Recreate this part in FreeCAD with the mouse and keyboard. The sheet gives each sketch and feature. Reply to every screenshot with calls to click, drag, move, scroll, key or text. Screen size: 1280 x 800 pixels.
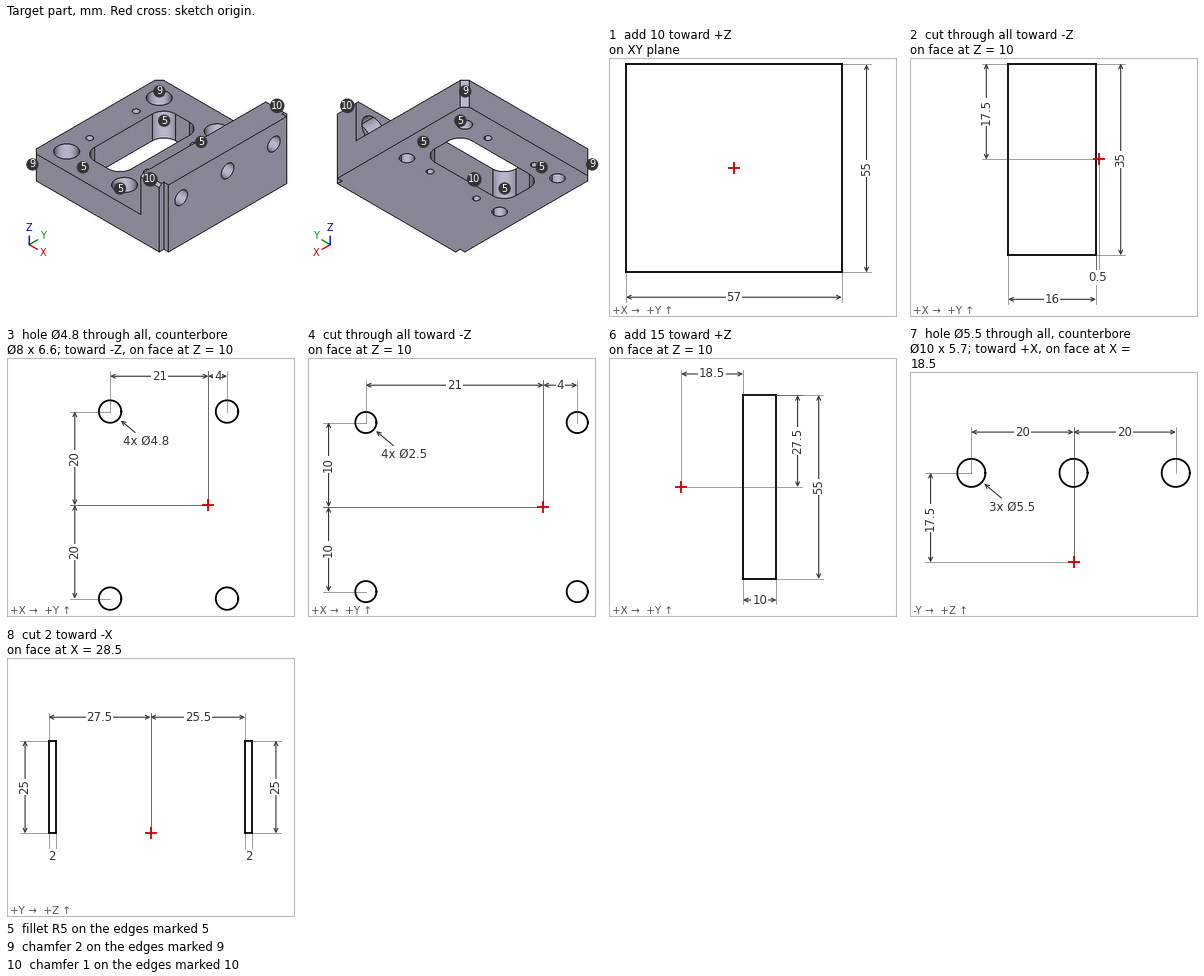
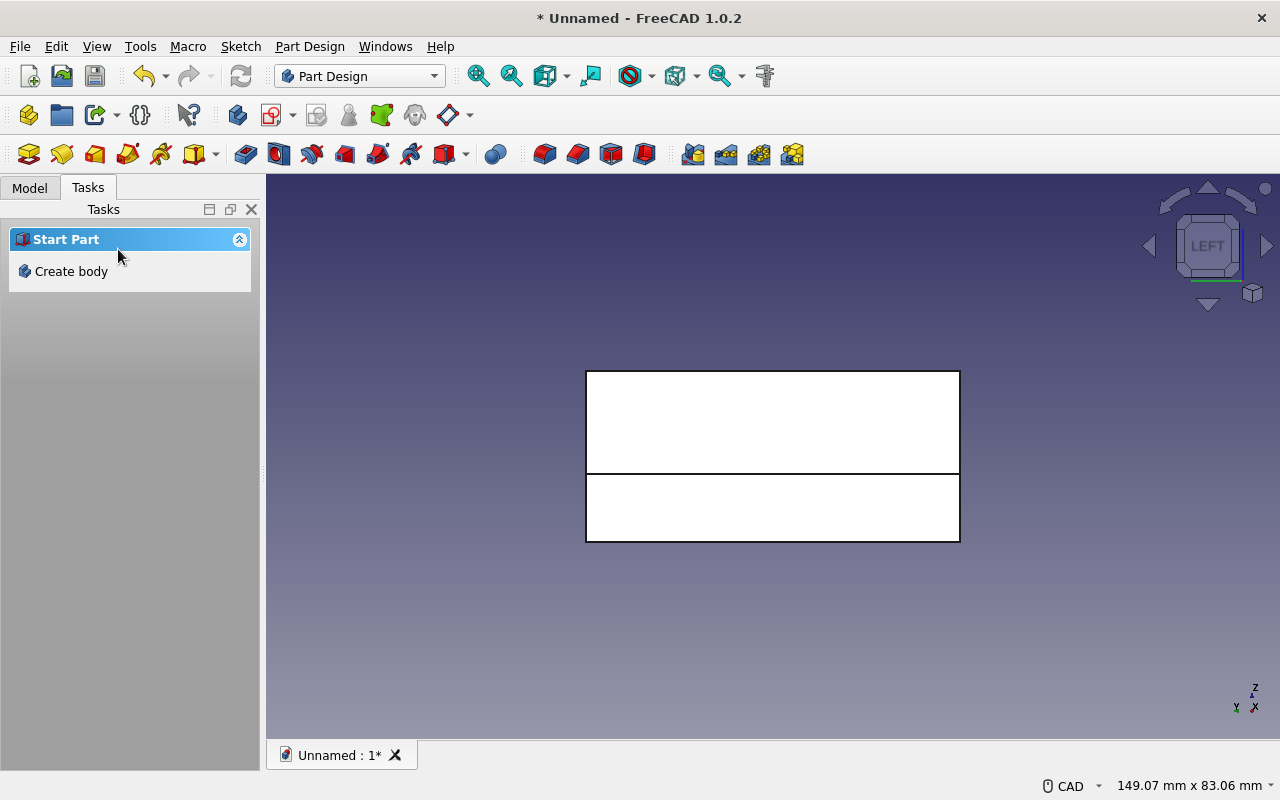
click(666, 421)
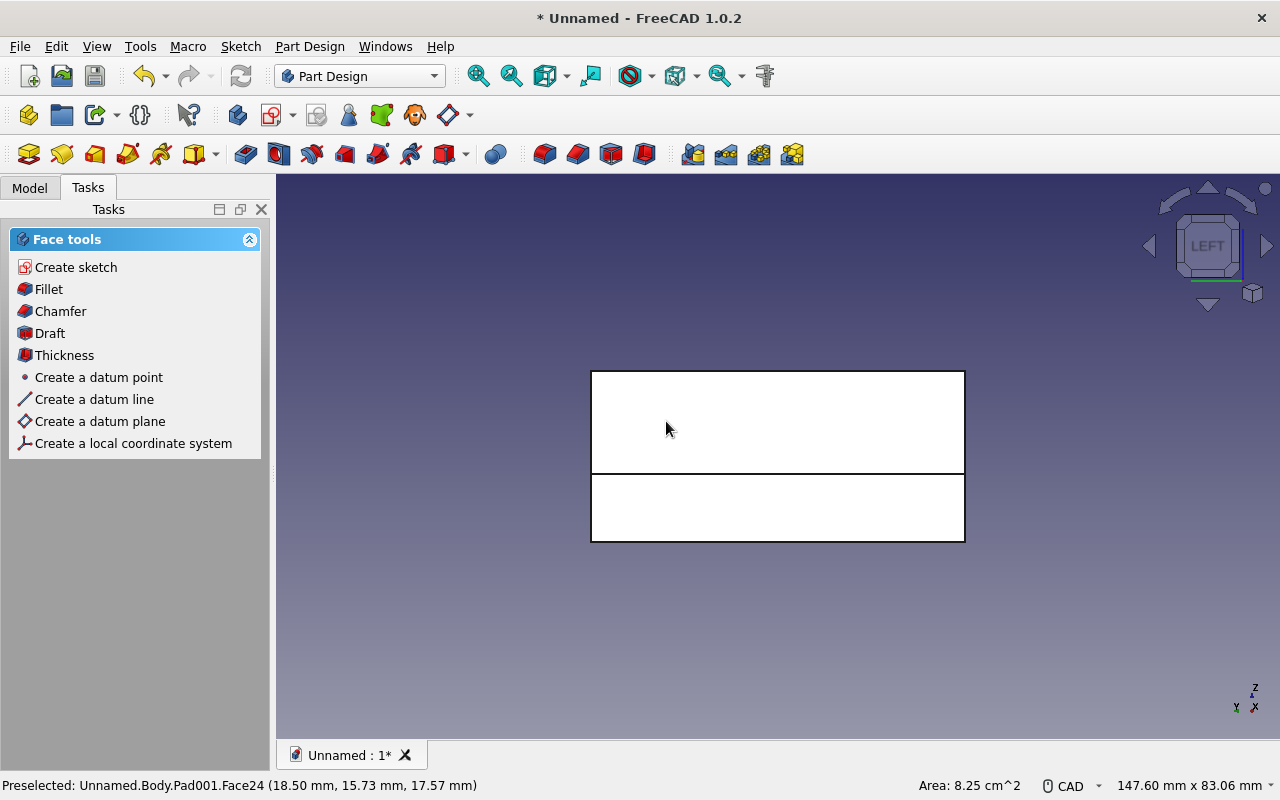
click(270, 116)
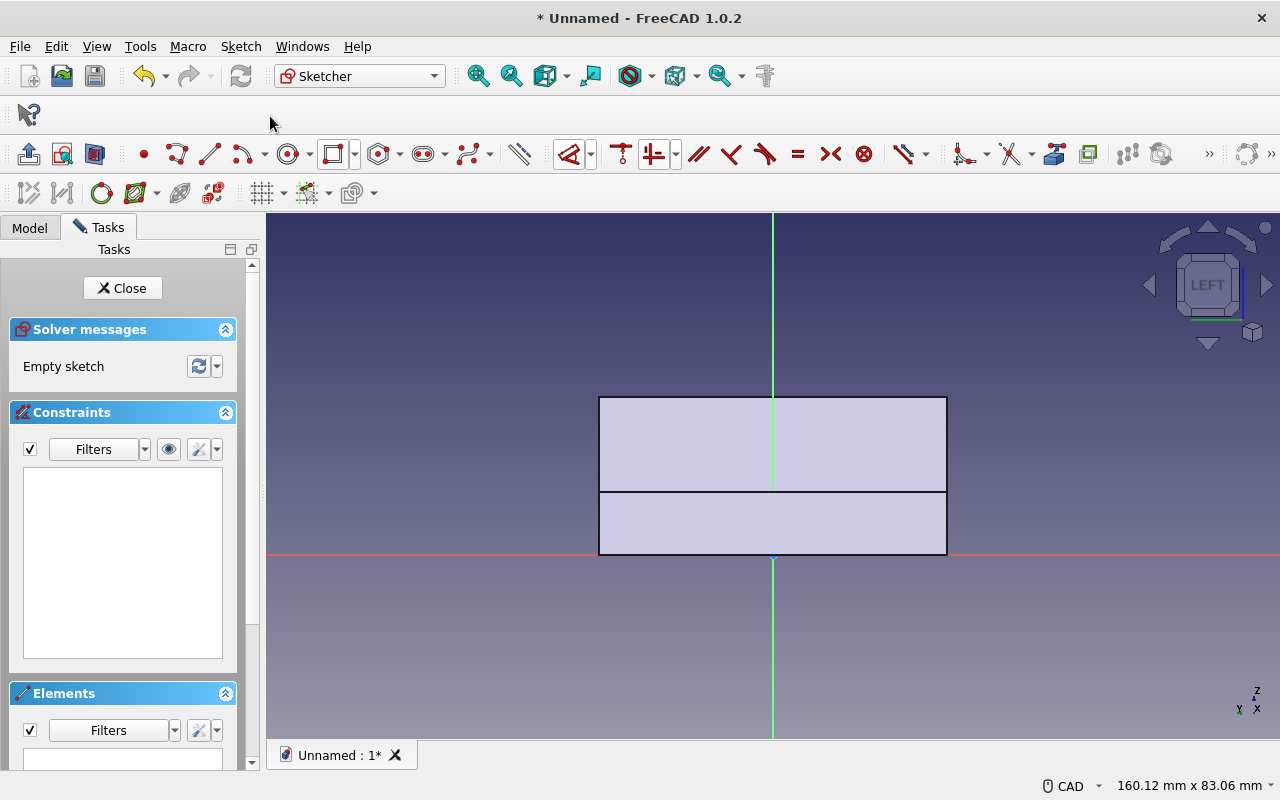
scroll(856, 509, up, 3)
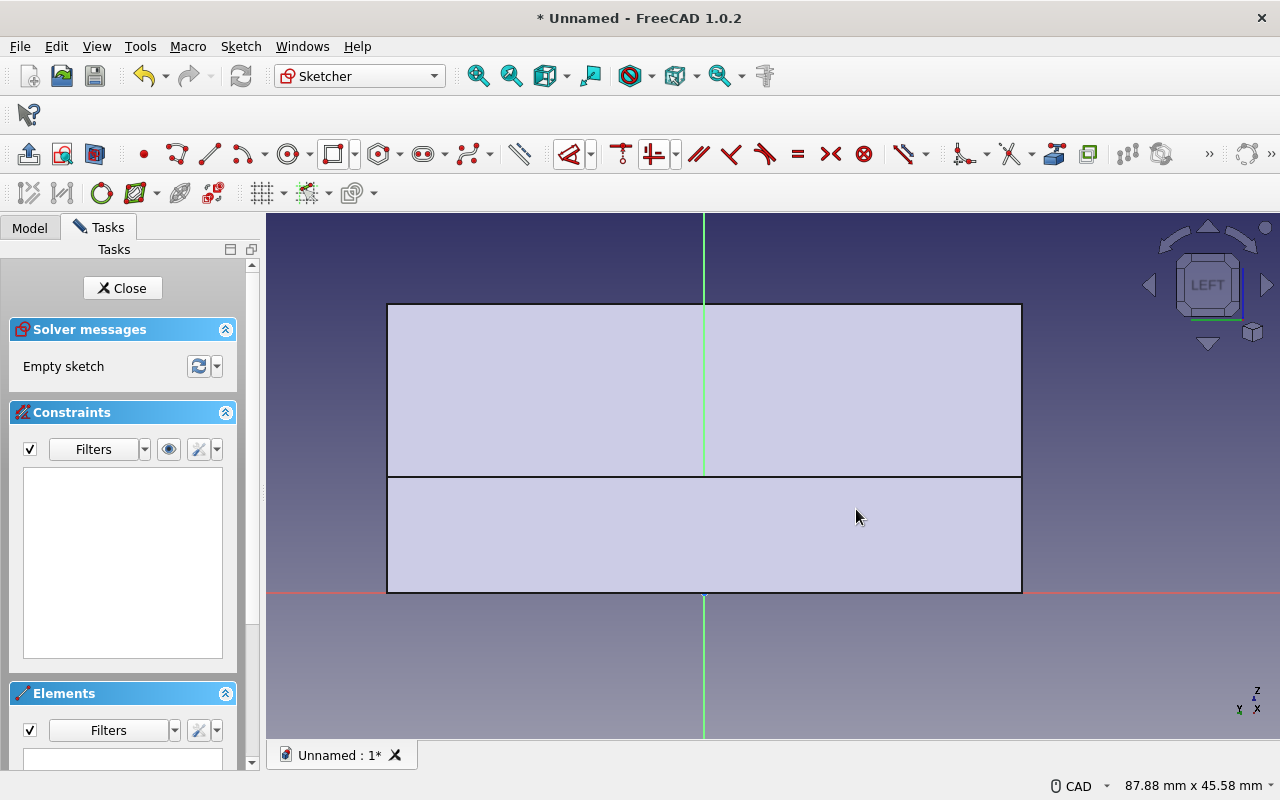
click(288, 154)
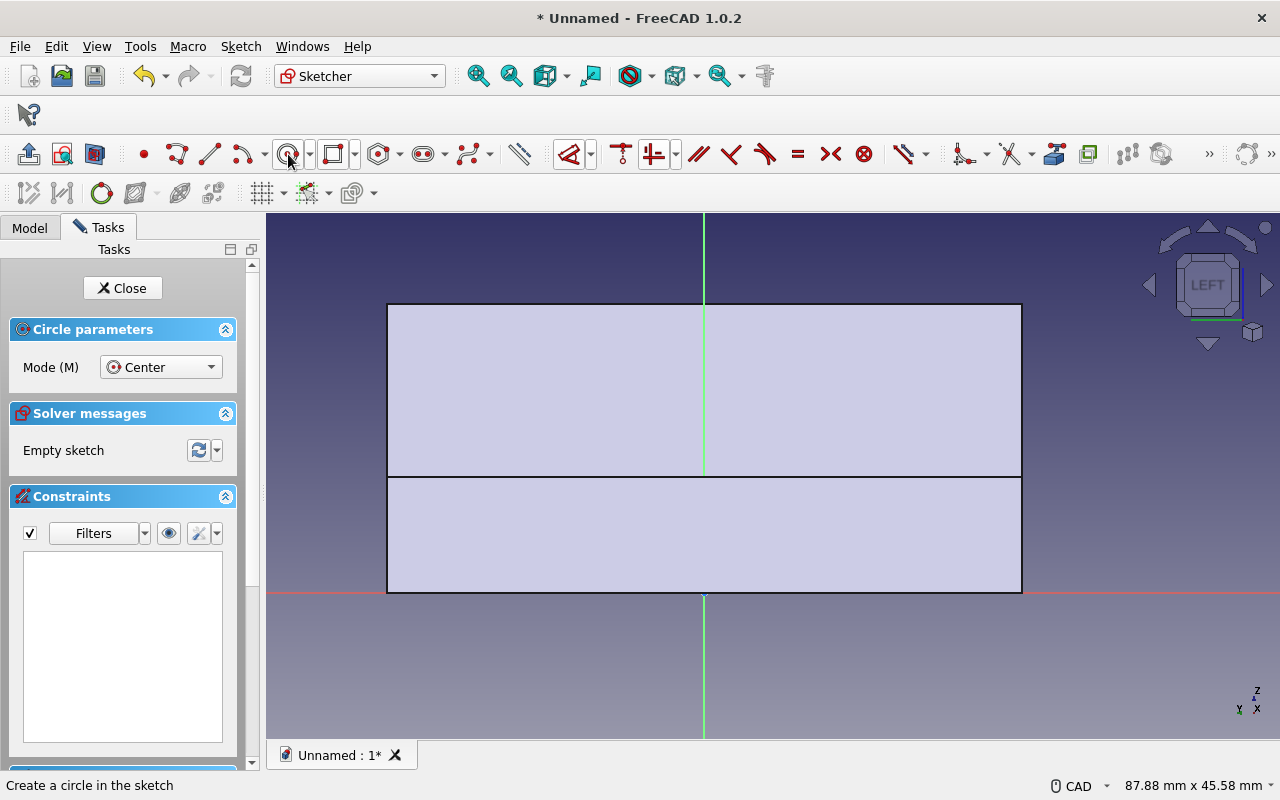
click(474, 391)
move(496, 368)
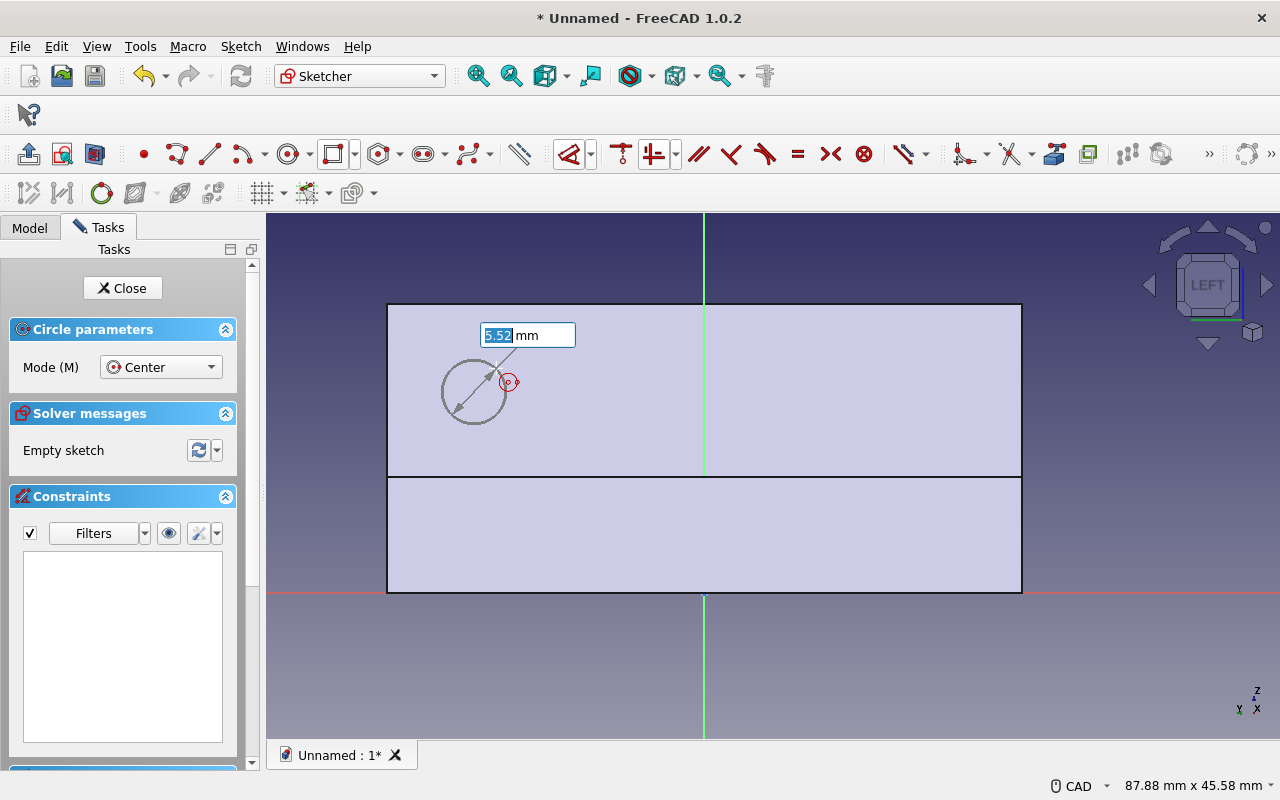
text(5.5)
key(Return)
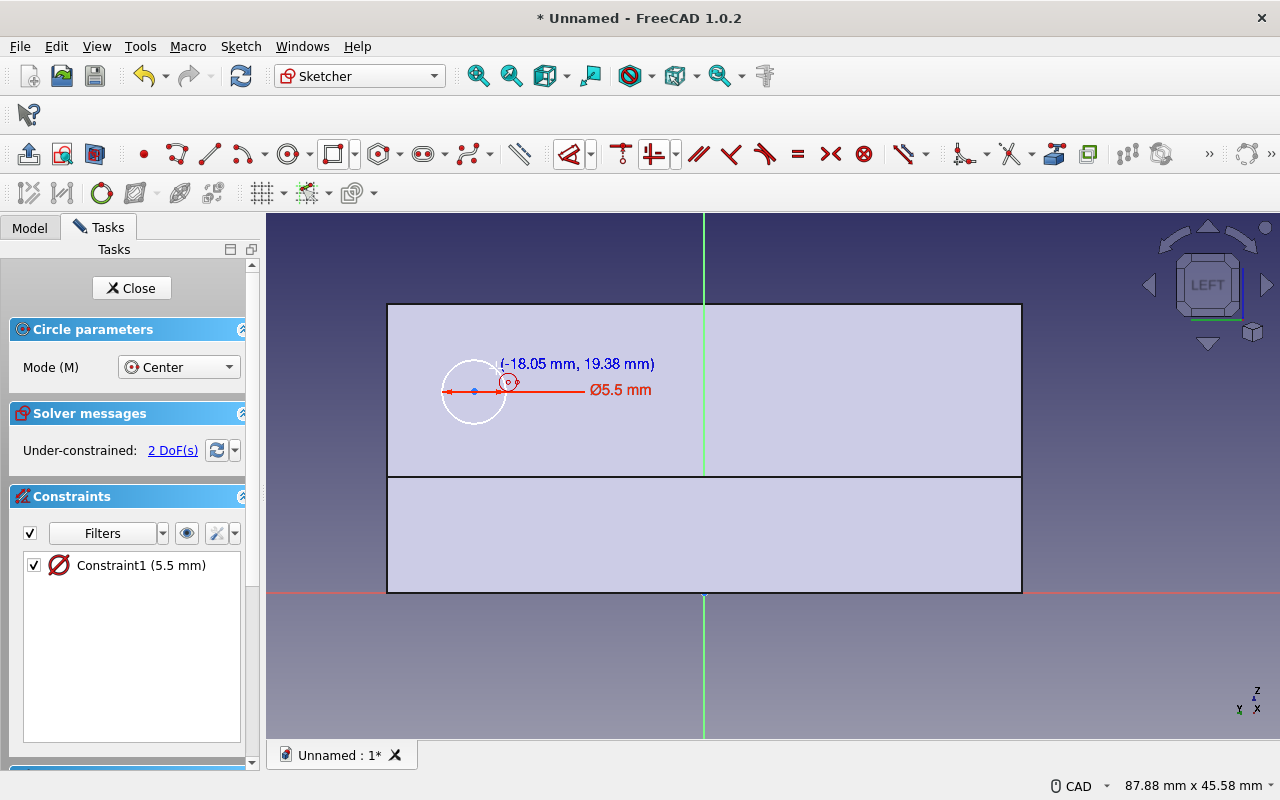
click(704, 391)
move(727, 368)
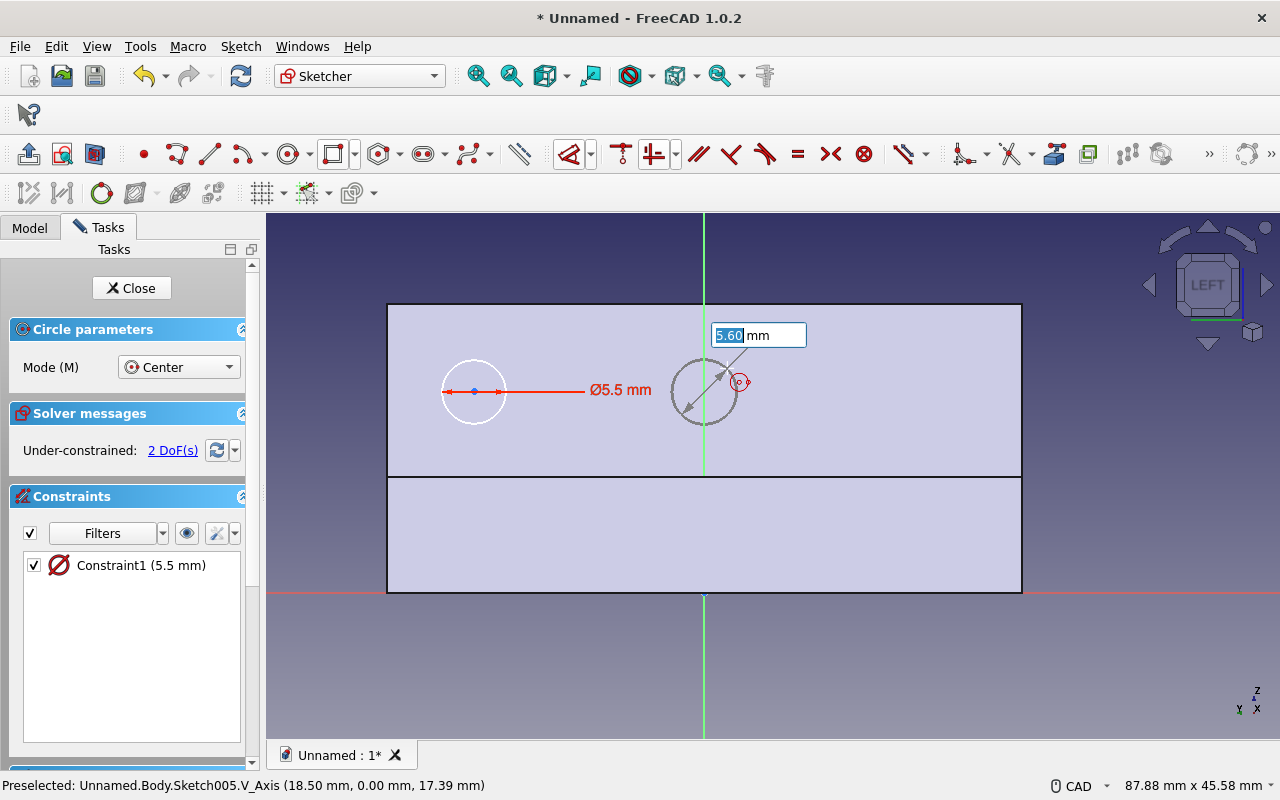
text(5.5)
key(Return)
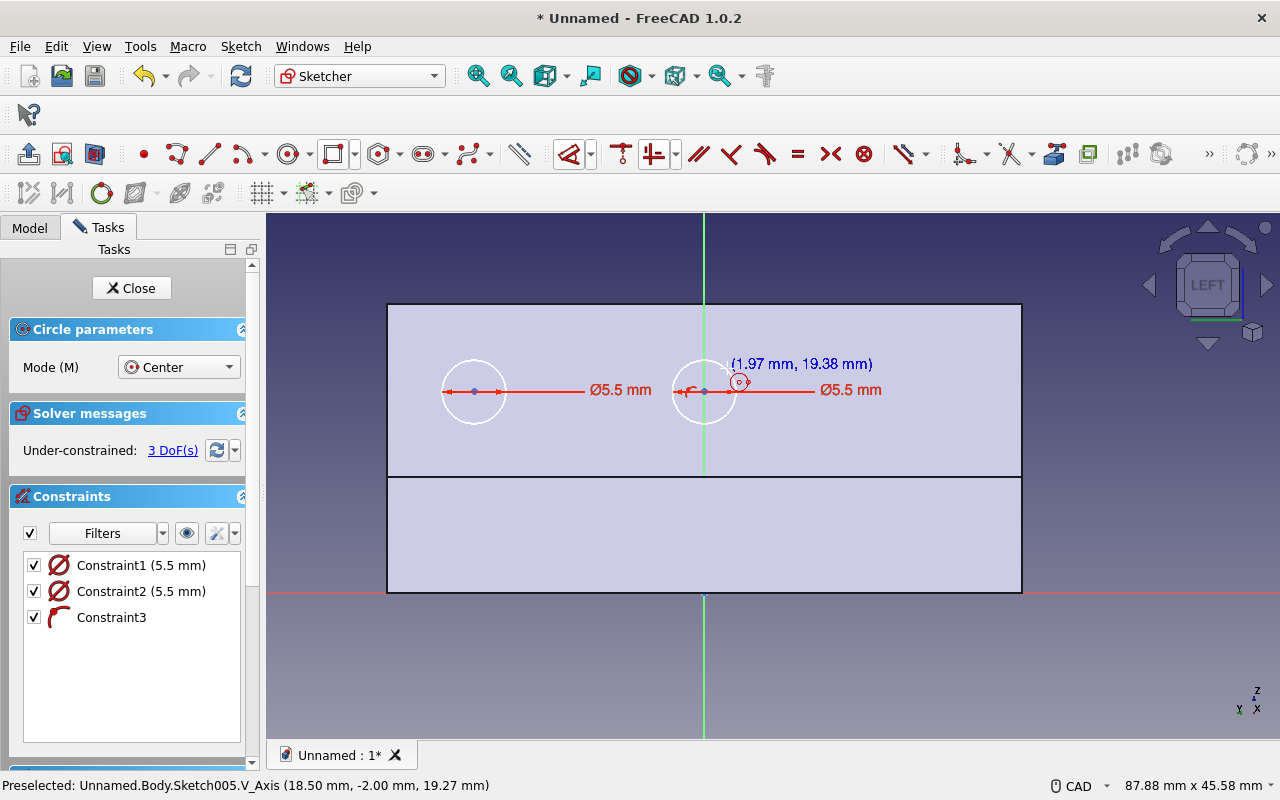
click(935, 391)
move(958, 368)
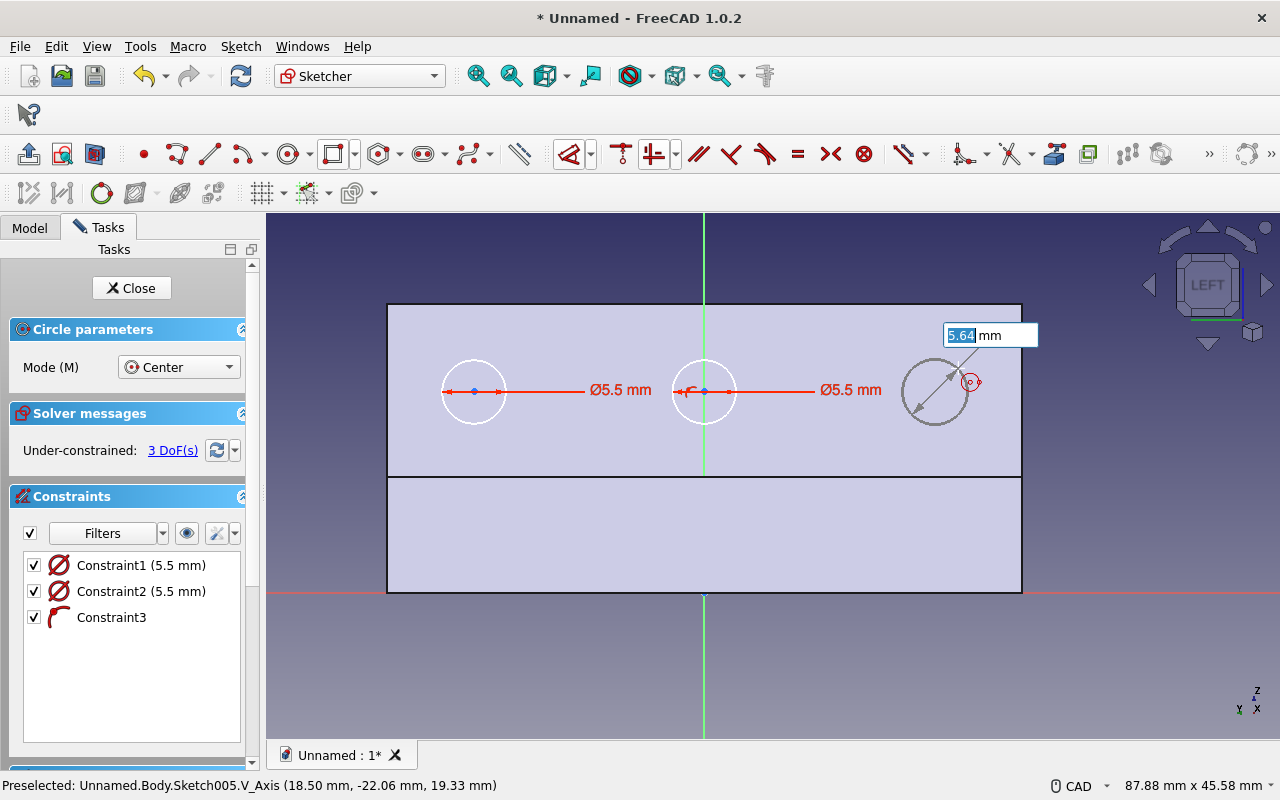
text(5.5)
key(Return)
key(Escape)